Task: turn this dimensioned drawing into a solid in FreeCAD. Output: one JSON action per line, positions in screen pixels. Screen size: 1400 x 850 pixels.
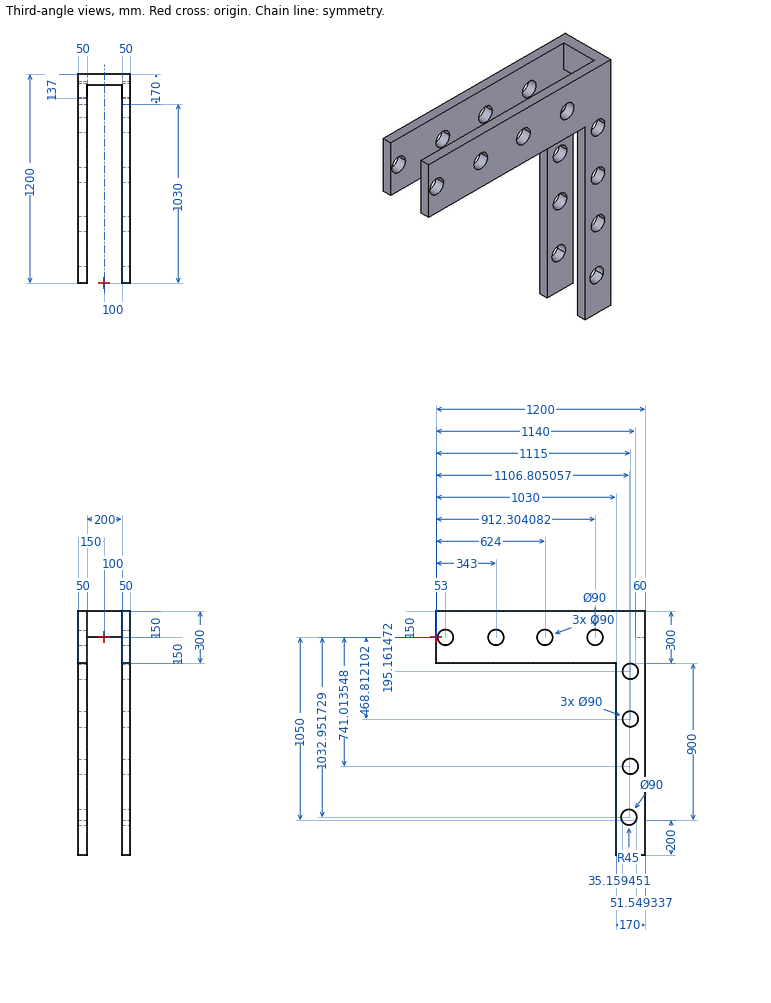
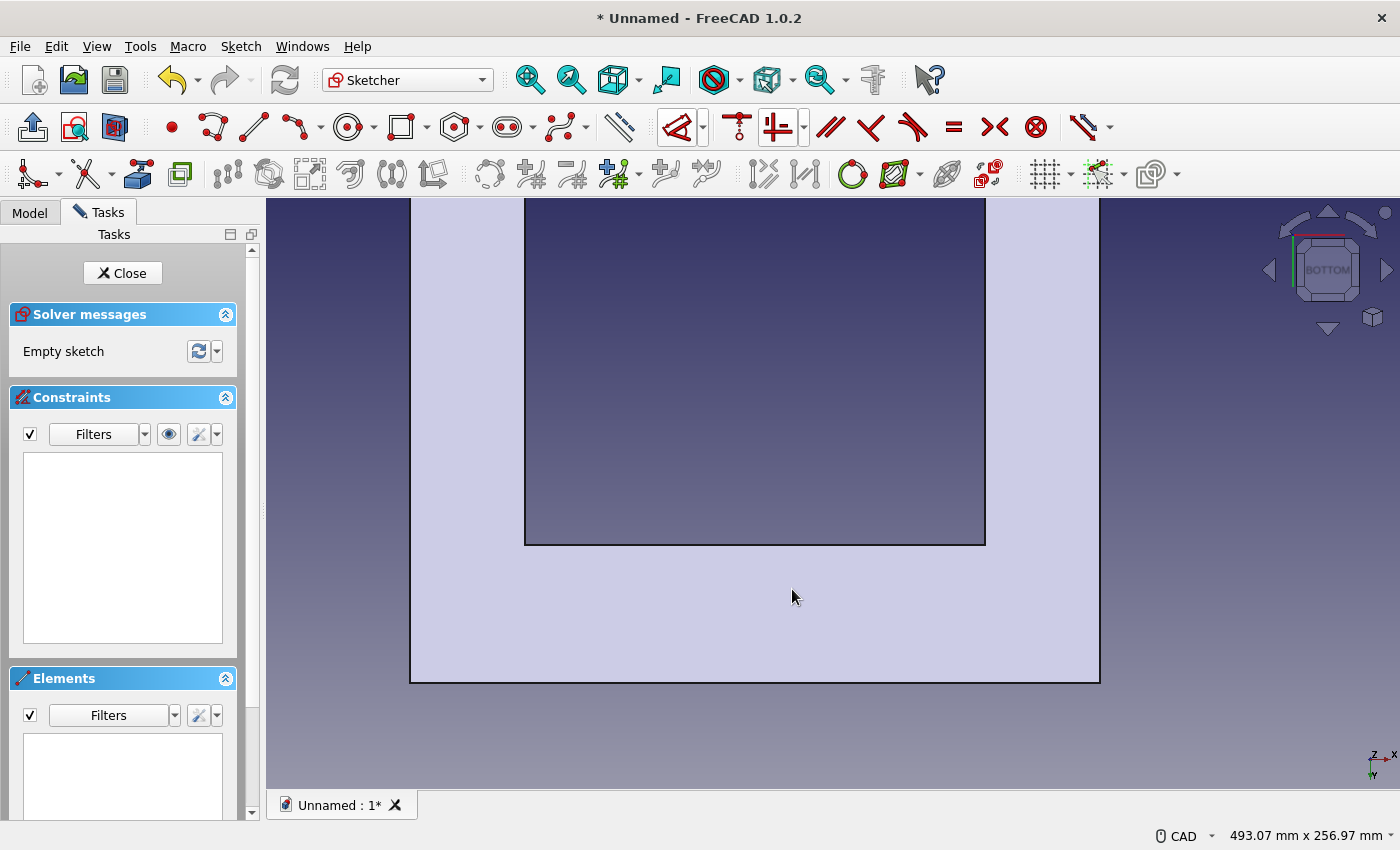
{"action": "left_click", "coordinate": [400, 128]}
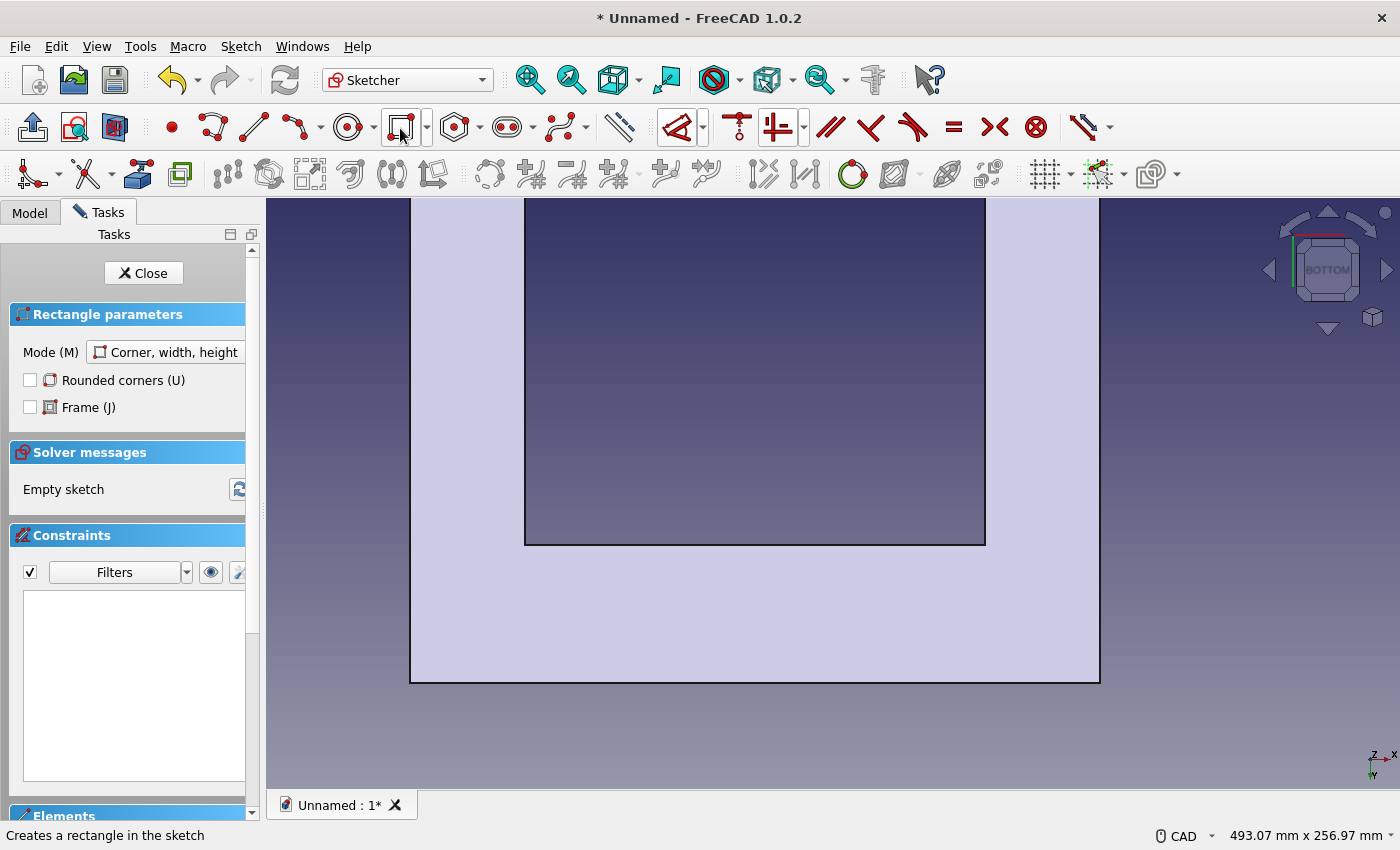
{"action": "left_click", "coordinate": [985, 292]}
{"action": "left_click", "coordinate": [1100, 683]}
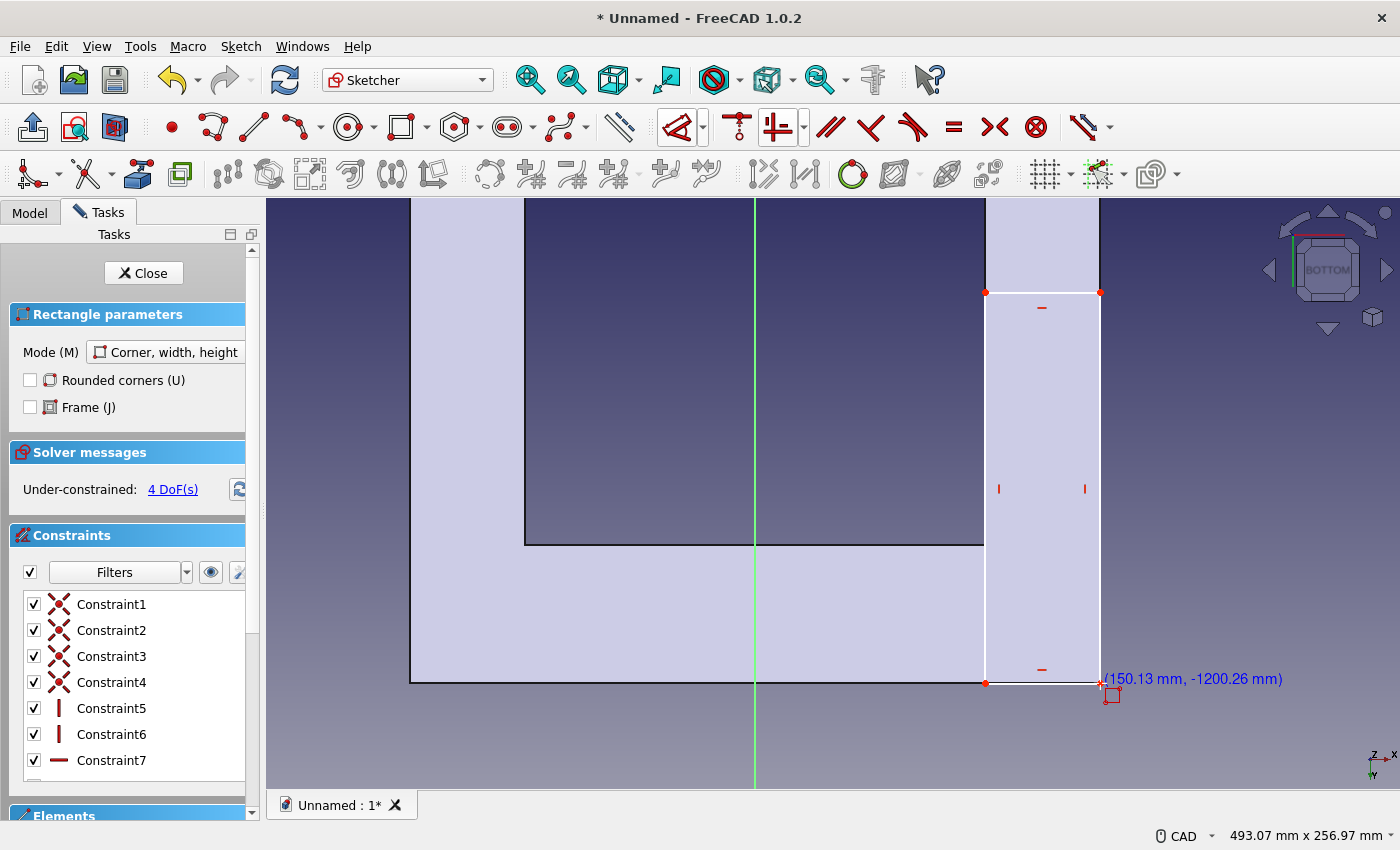
{"action": "left_click", "coordinate": [410, 292]}
{"action": "left_click", "coordinate": [525, 683]}
{"action": "key", "text": "Escape"}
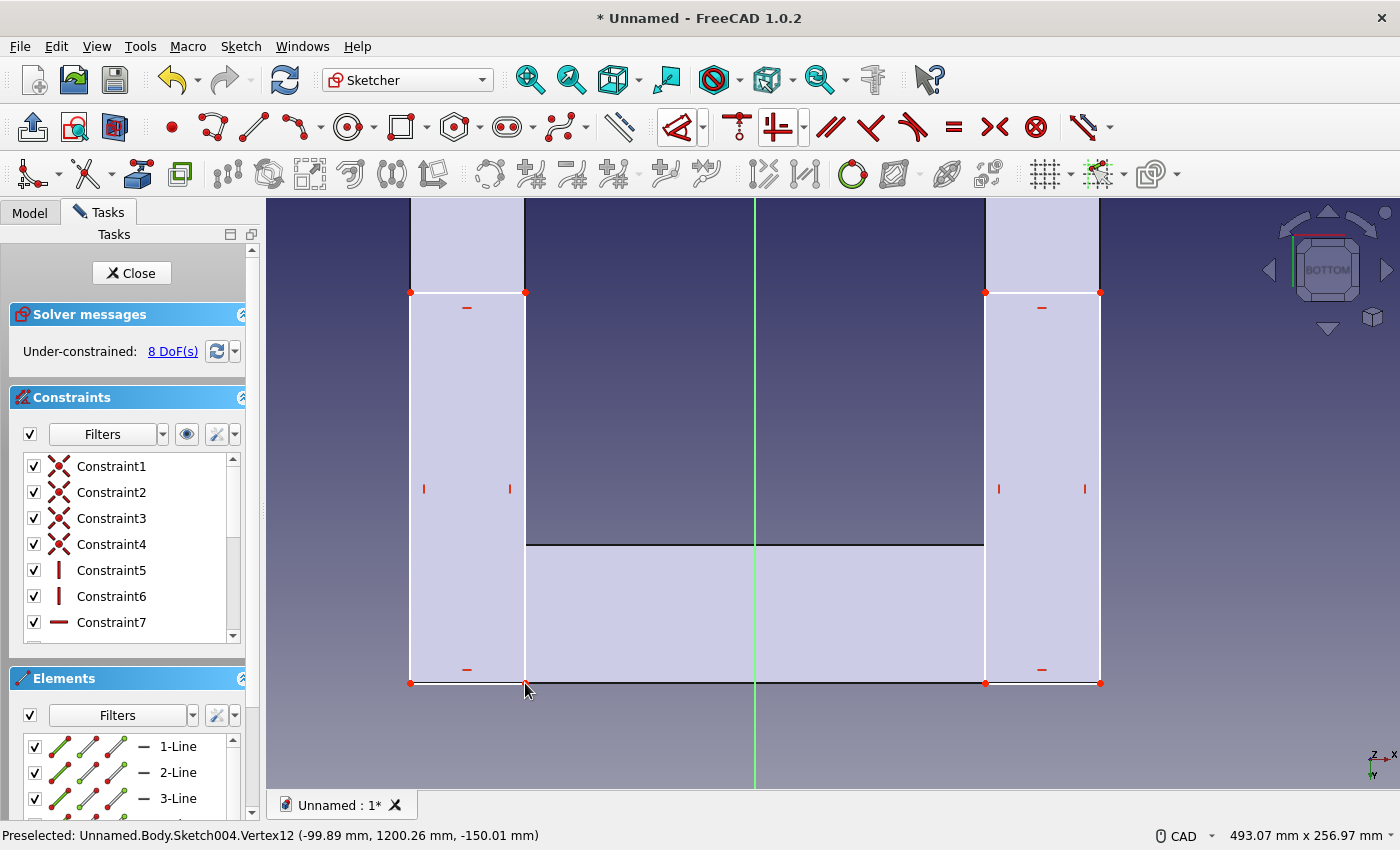
{"action": "left_click", "coordinate": [1100, 293]}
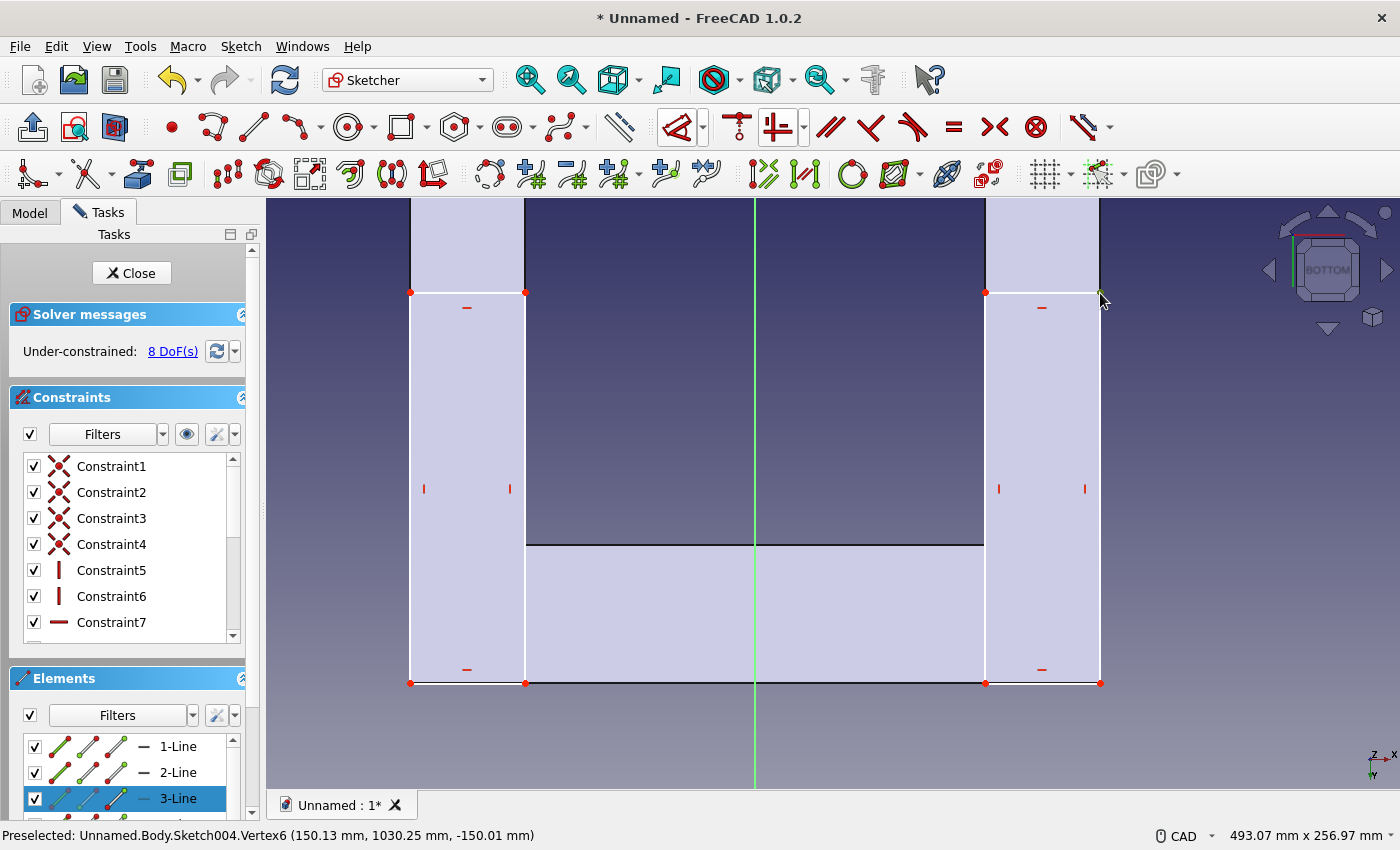
{"action": "left_click", "coordinate": [410, 293]}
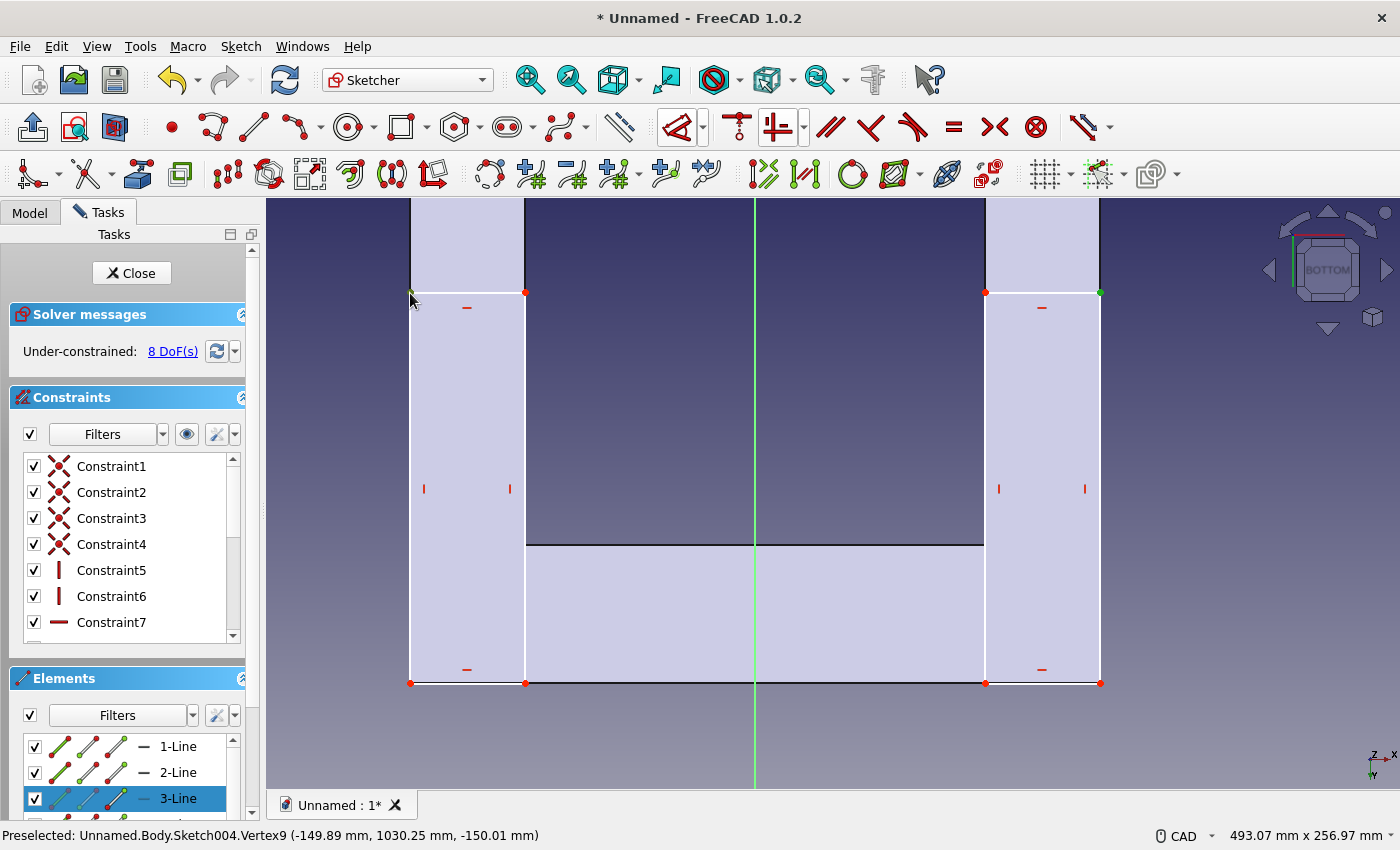
{"action": "left_click", "coordinate": [755, 723]}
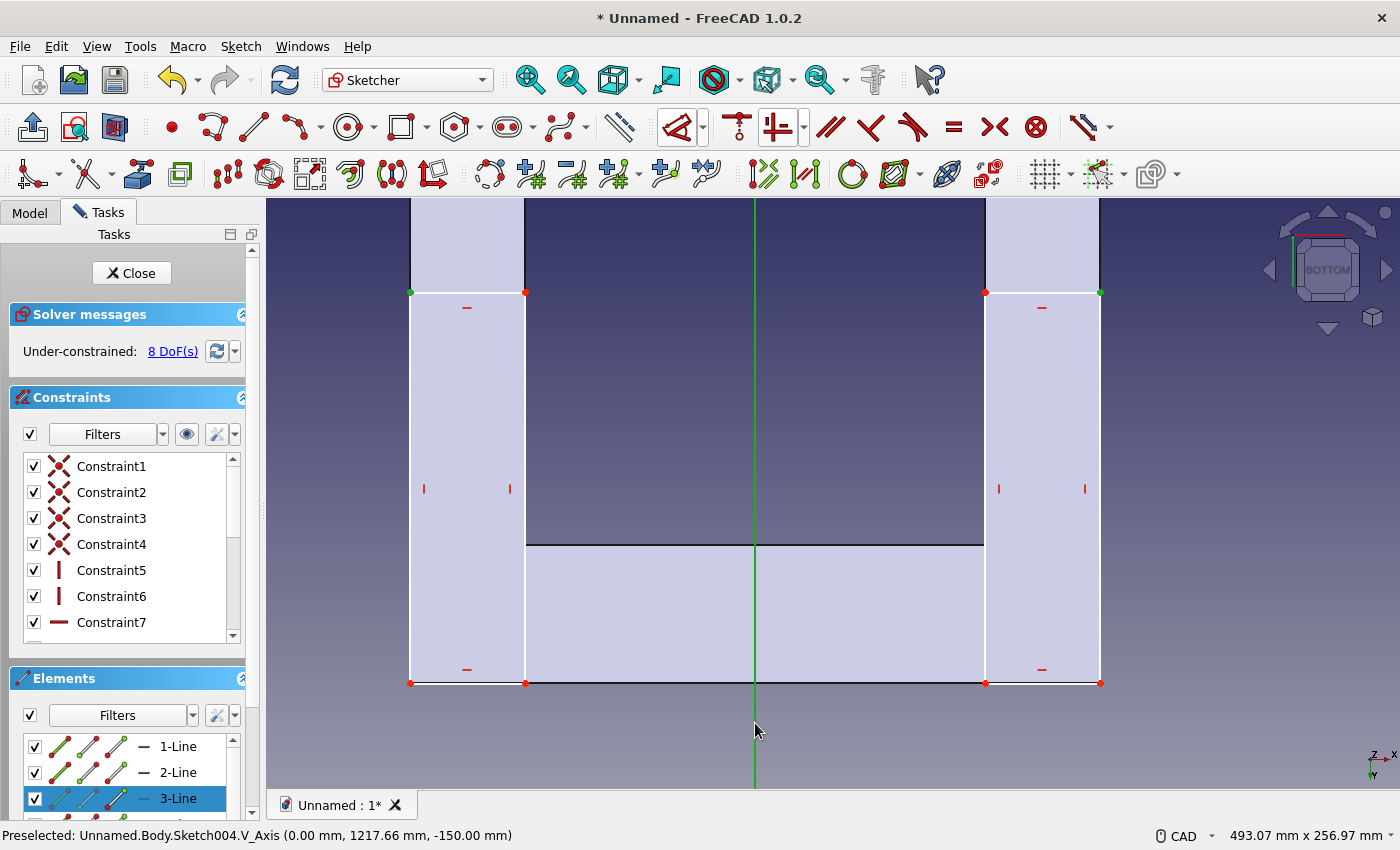
{"action": "left_click", "coordinate": [995, 128]}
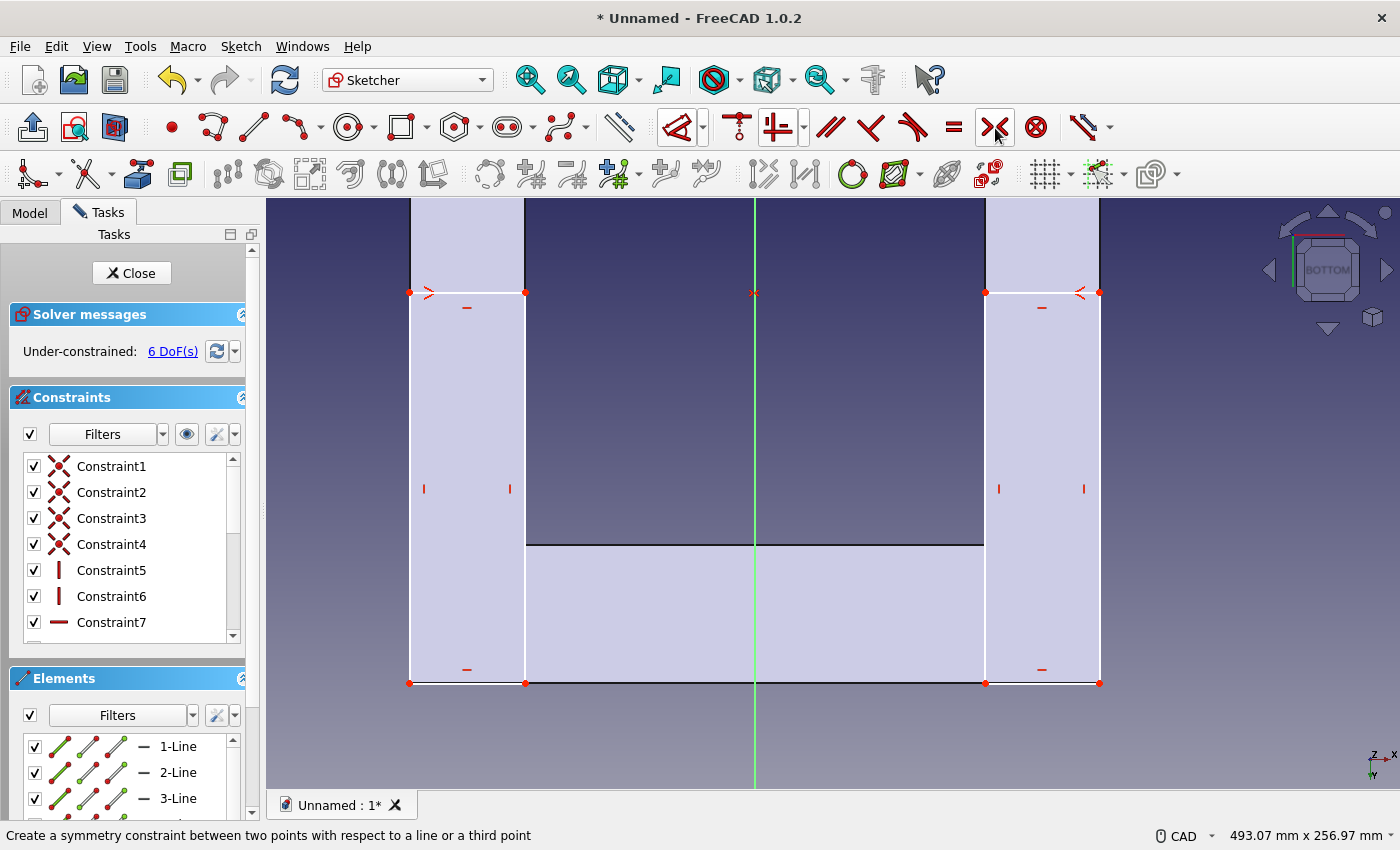
{"action": "left_click", "coordinate": [985, 684]}